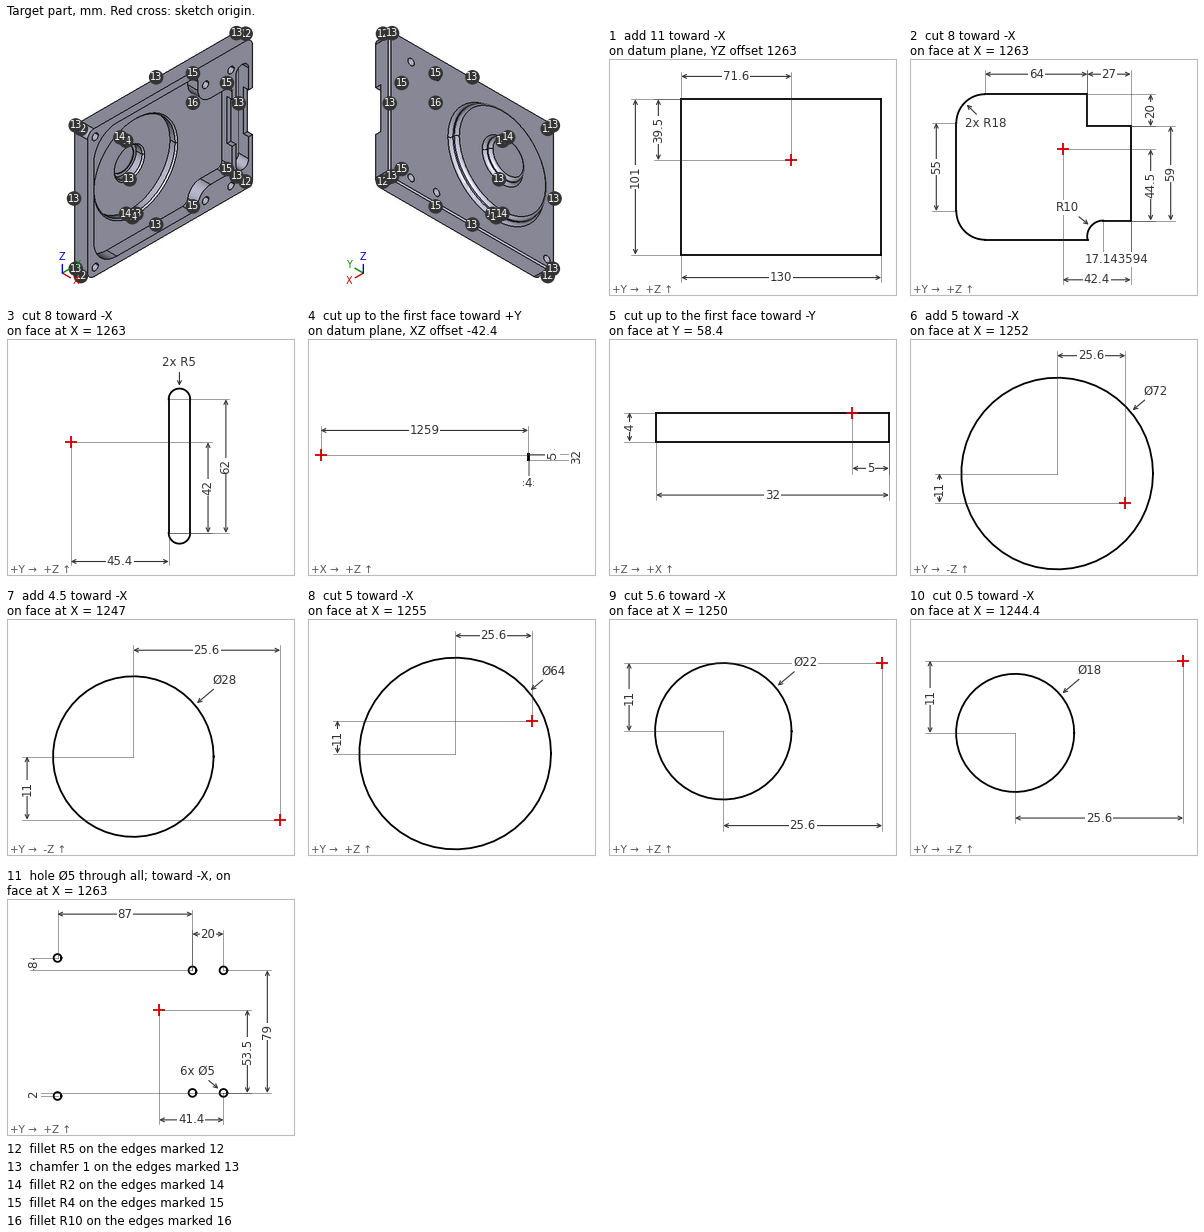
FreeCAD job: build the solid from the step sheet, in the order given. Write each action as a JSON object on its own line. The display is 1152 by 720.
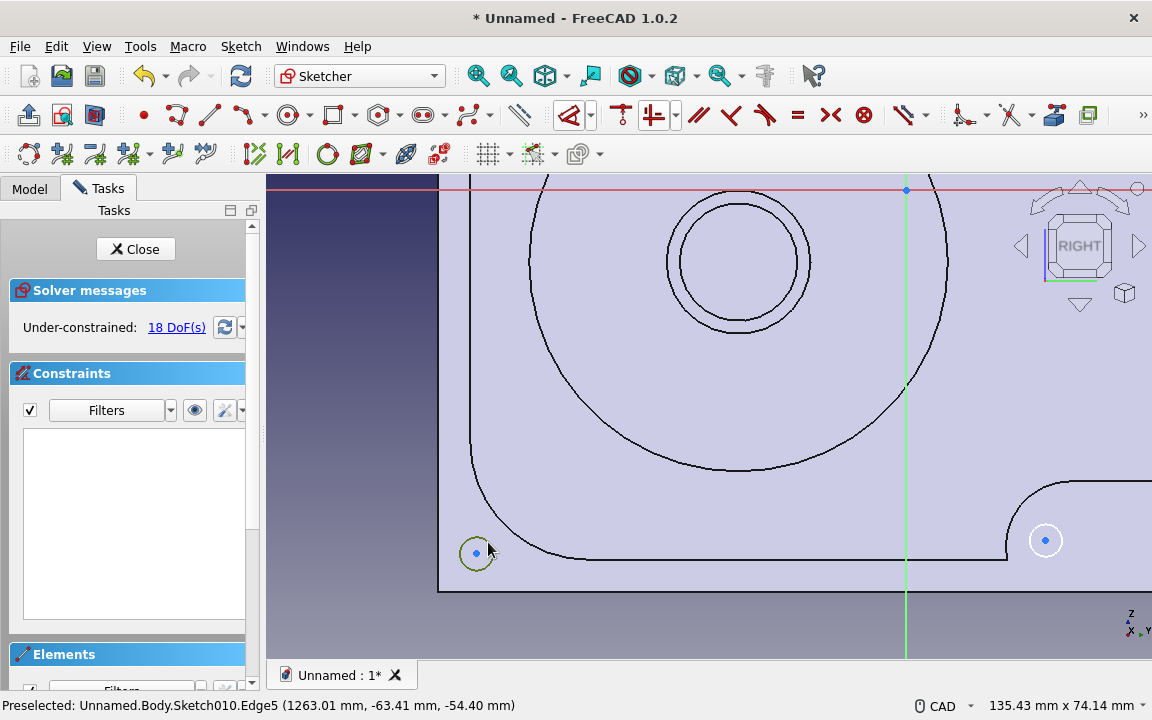
{"action": "scroll", "coordinate": [488, 543], "scroll_direction": "down", "scroll_amount": 4}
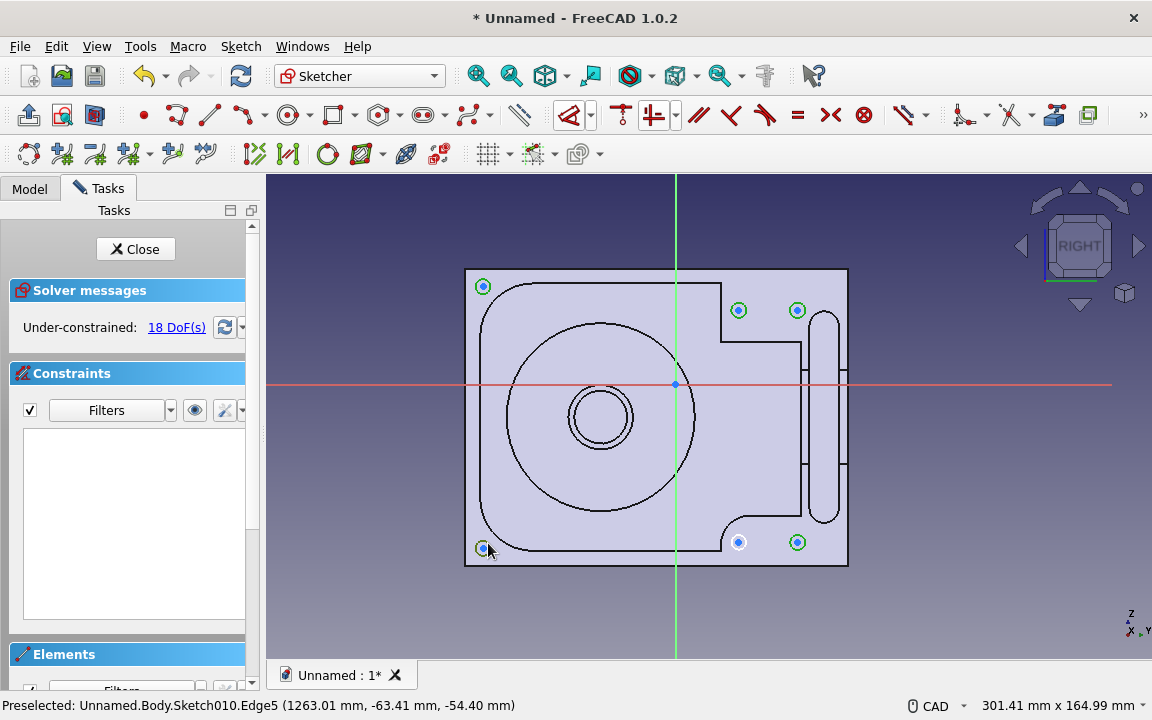
{"action": "scroll", "coordinate": [744, 537], "scroll_direction": "up", "scroll_amount": 4}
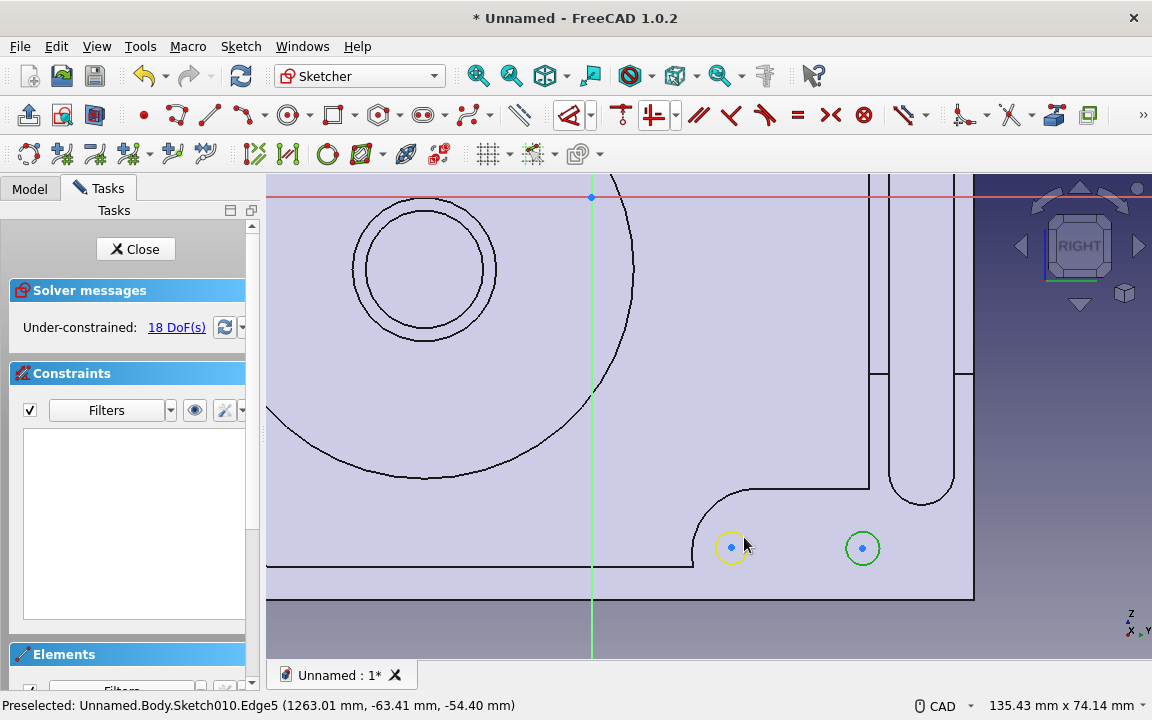
{"action": "left_click", "coordinate": [743, 537]}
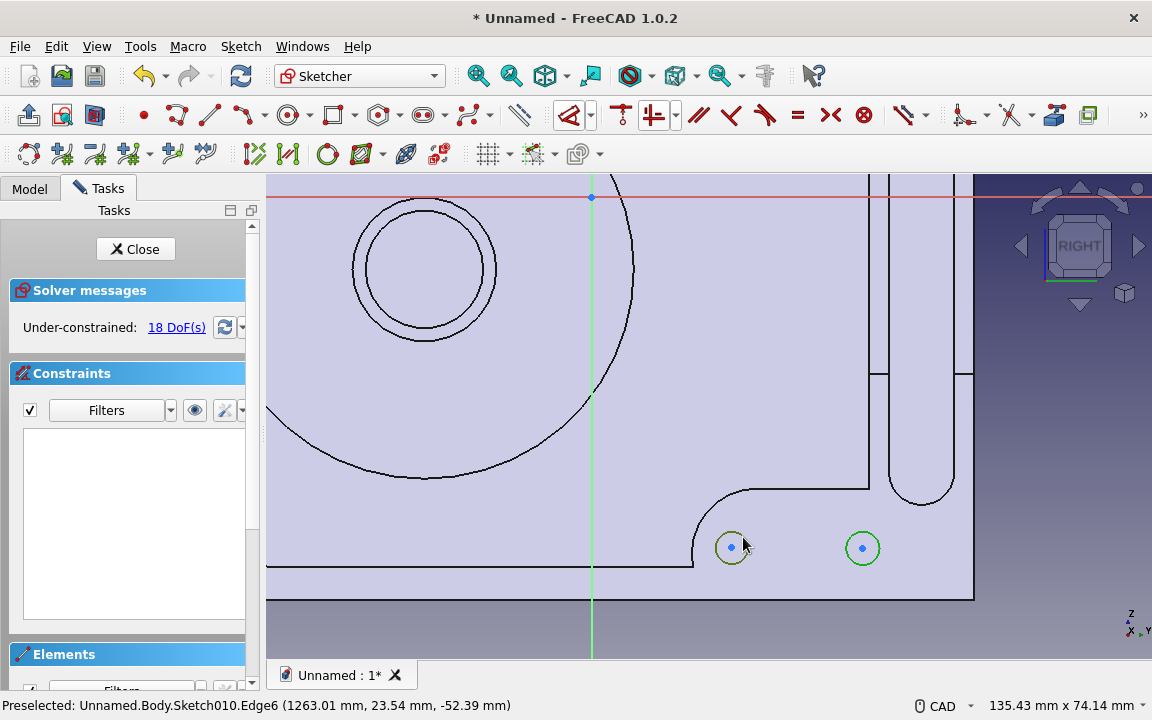
{"action": "left_click", "coordinate": [798, 116]}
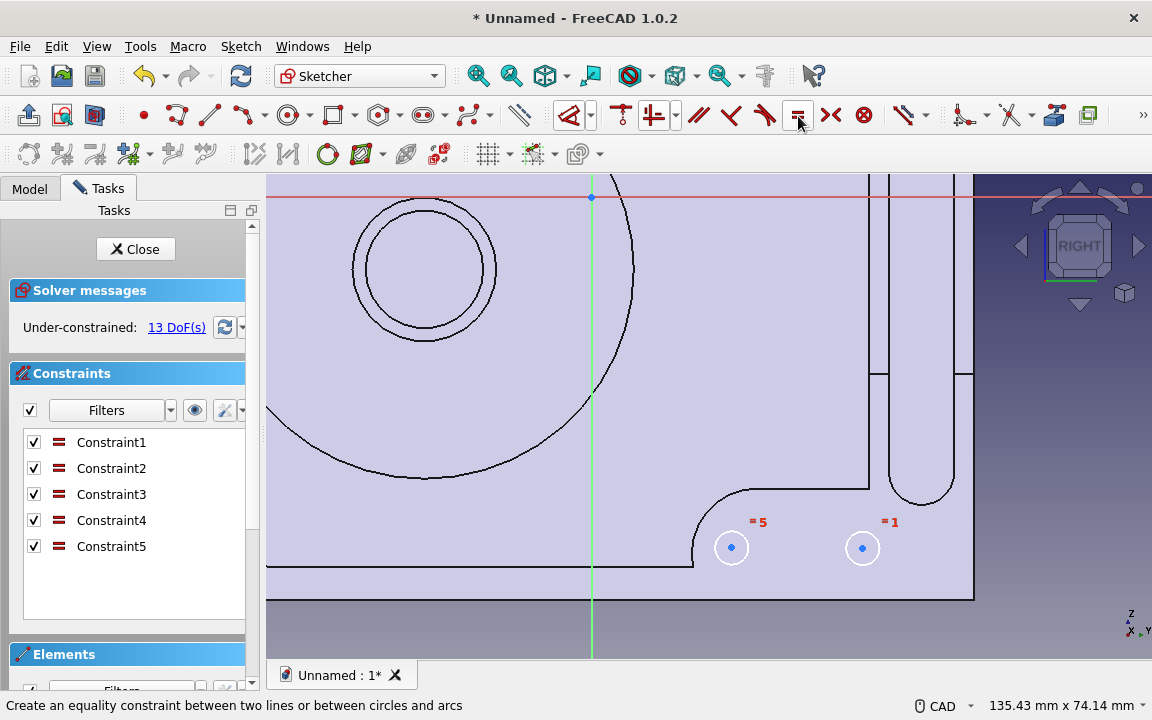
{"action": "left_click", "coordinate": [863, 548]}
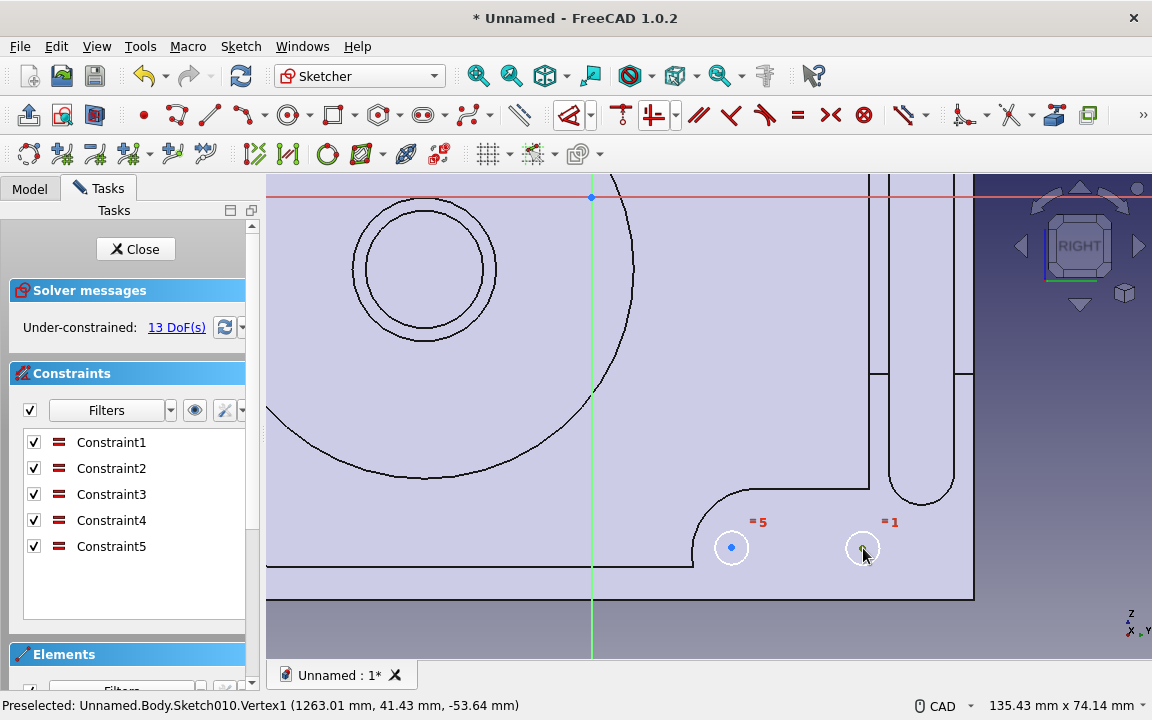
{"action": "scroll", "coordinate": [745, 537], "scroll_direction": "down", "scroll_amount": 4}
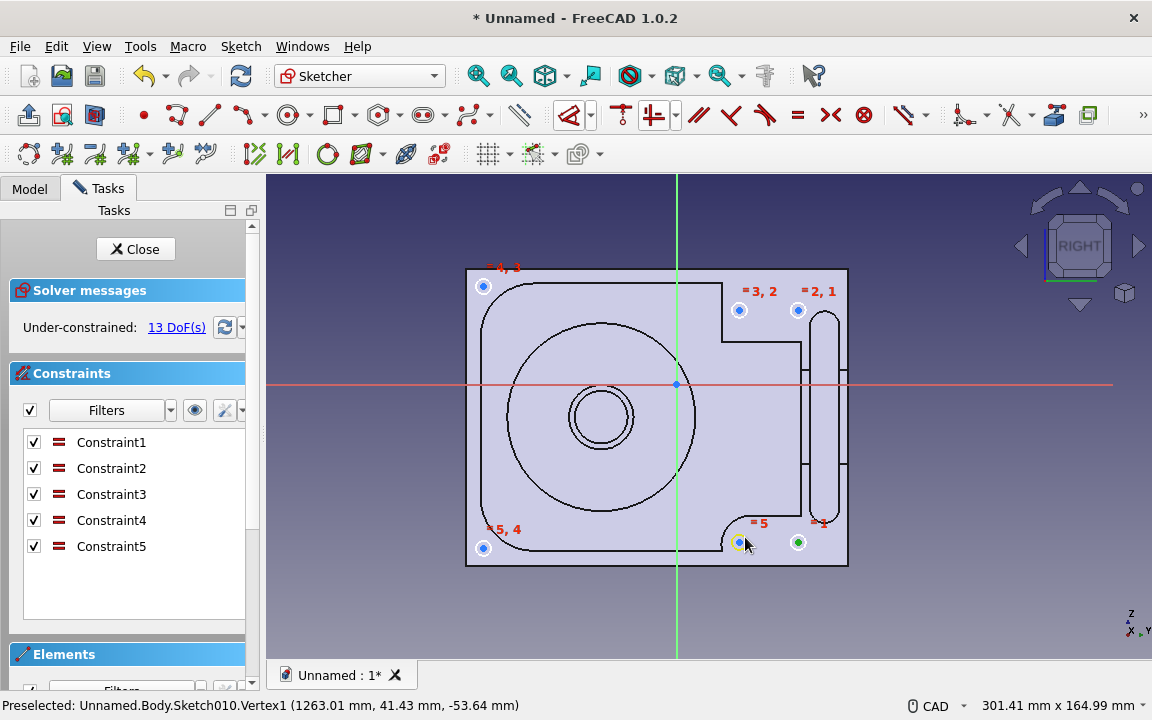
{"action": "left_click", "coordinate": [798, 310]}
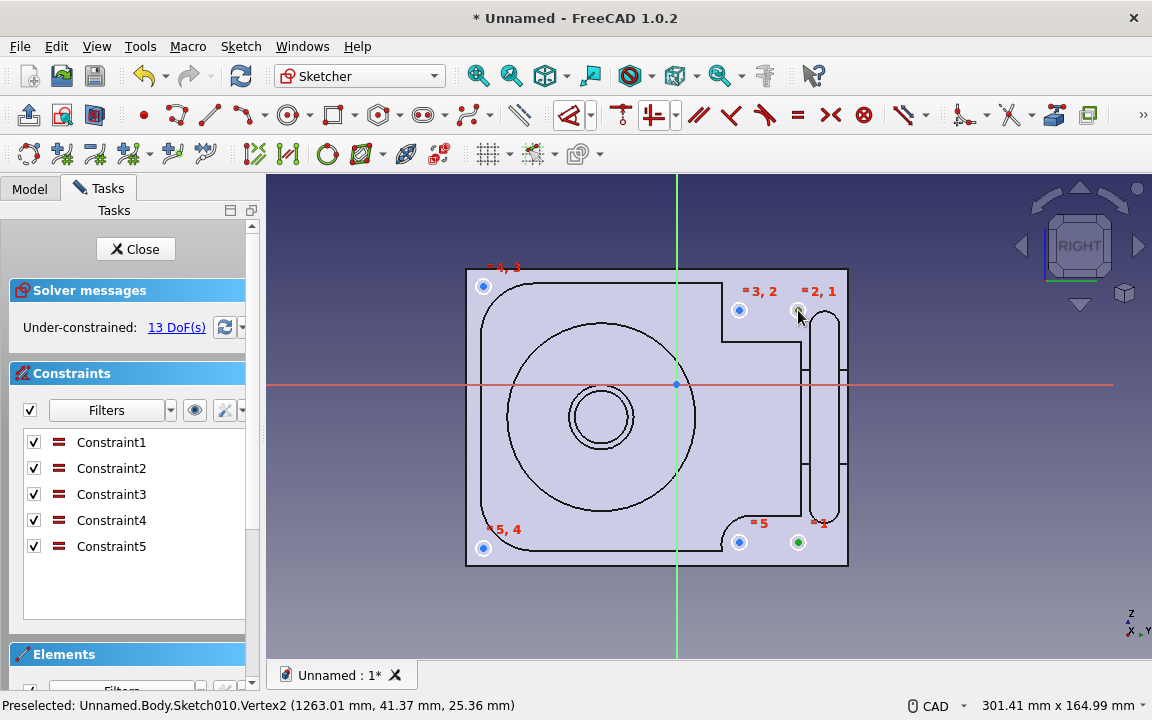
{"action": "key", "text": "v"}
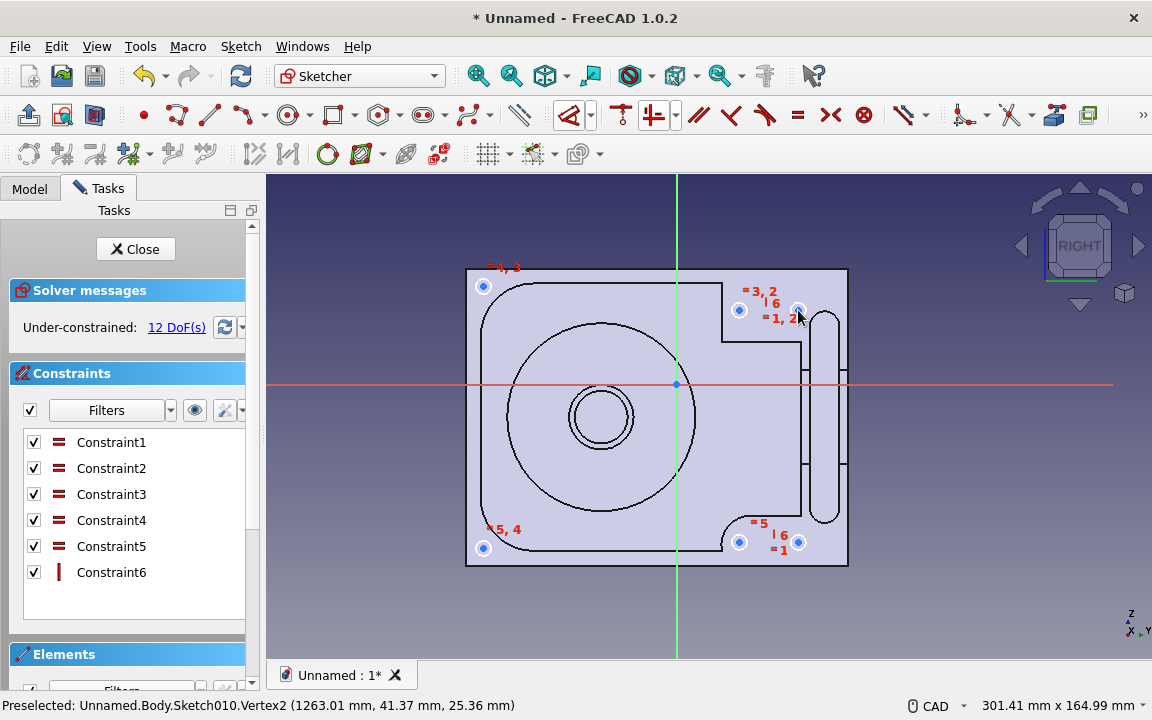
{"action": "left_click", "coordinate": [798, 310]}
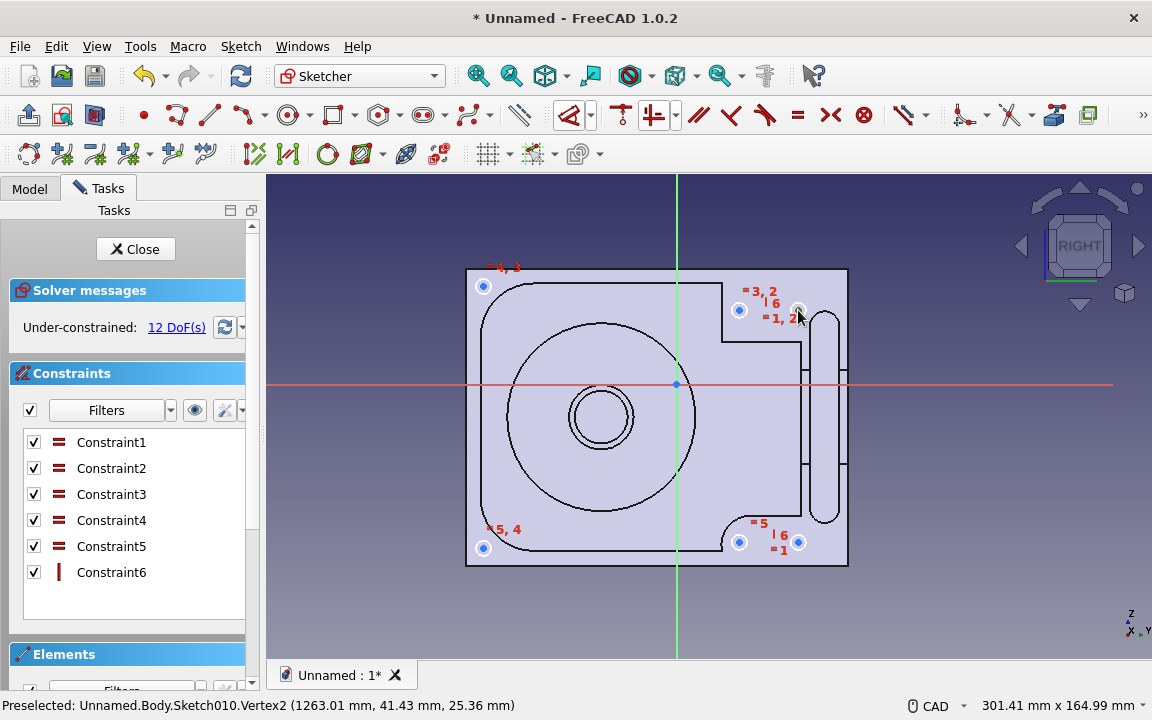
{"action": "left_click", "coordinate": [739, 310]}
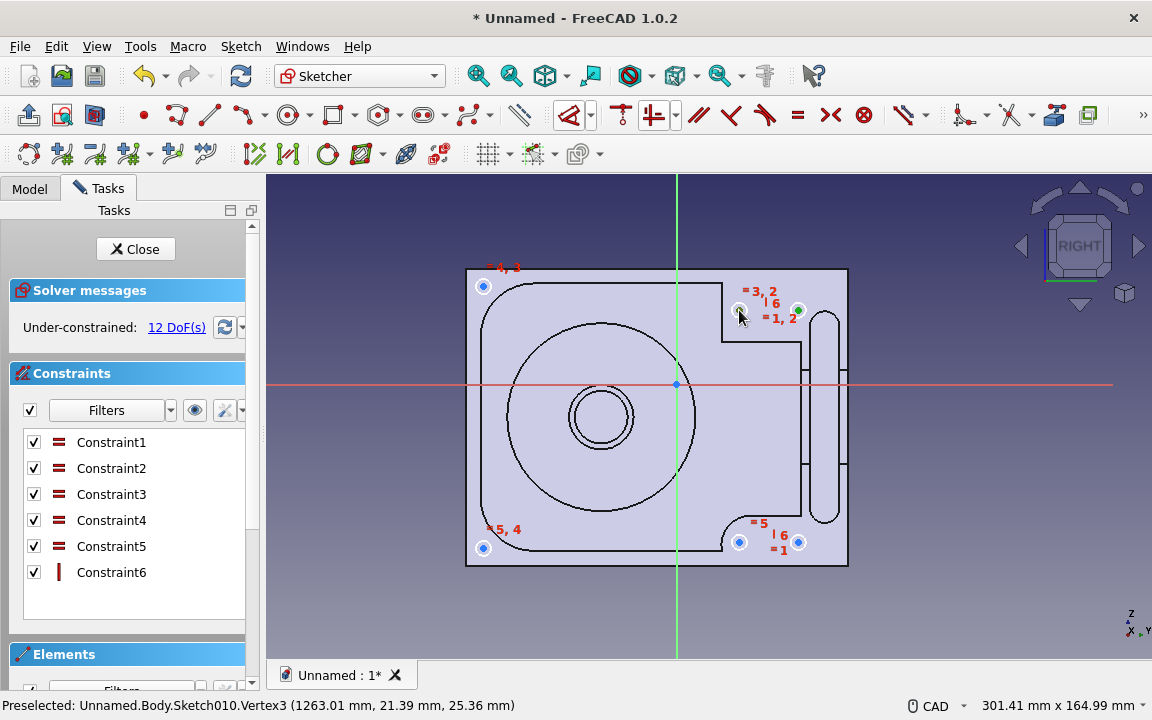
{"action": "left_click", "coordinate": [676, 116]}